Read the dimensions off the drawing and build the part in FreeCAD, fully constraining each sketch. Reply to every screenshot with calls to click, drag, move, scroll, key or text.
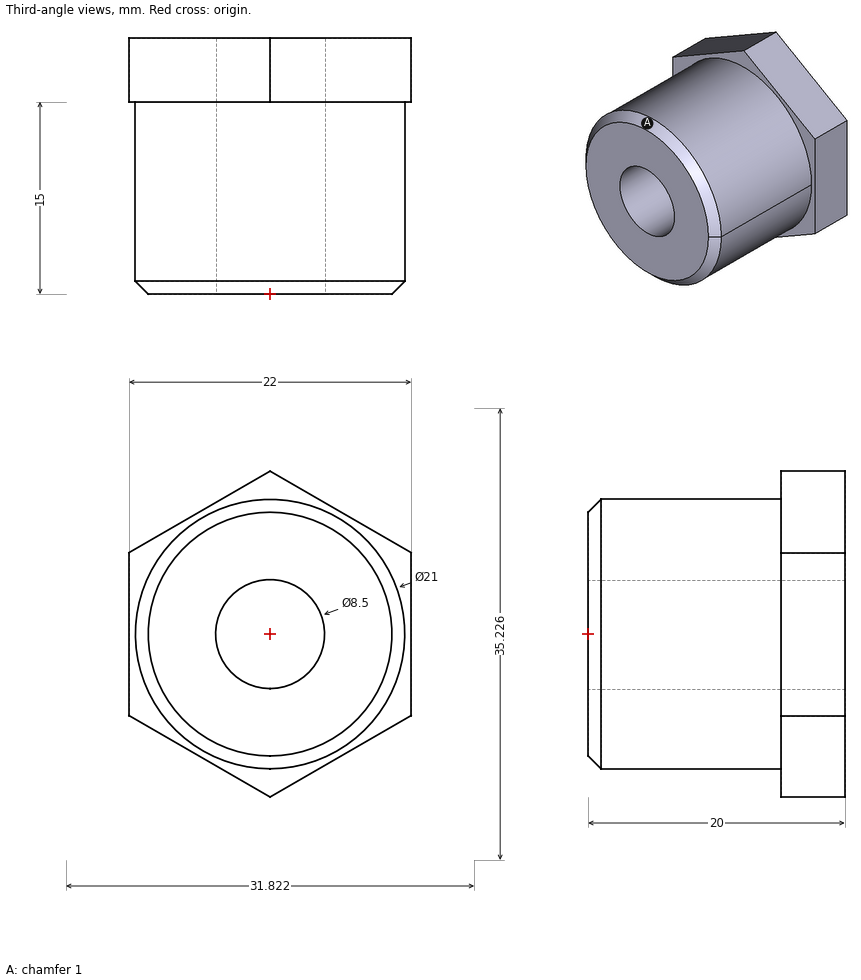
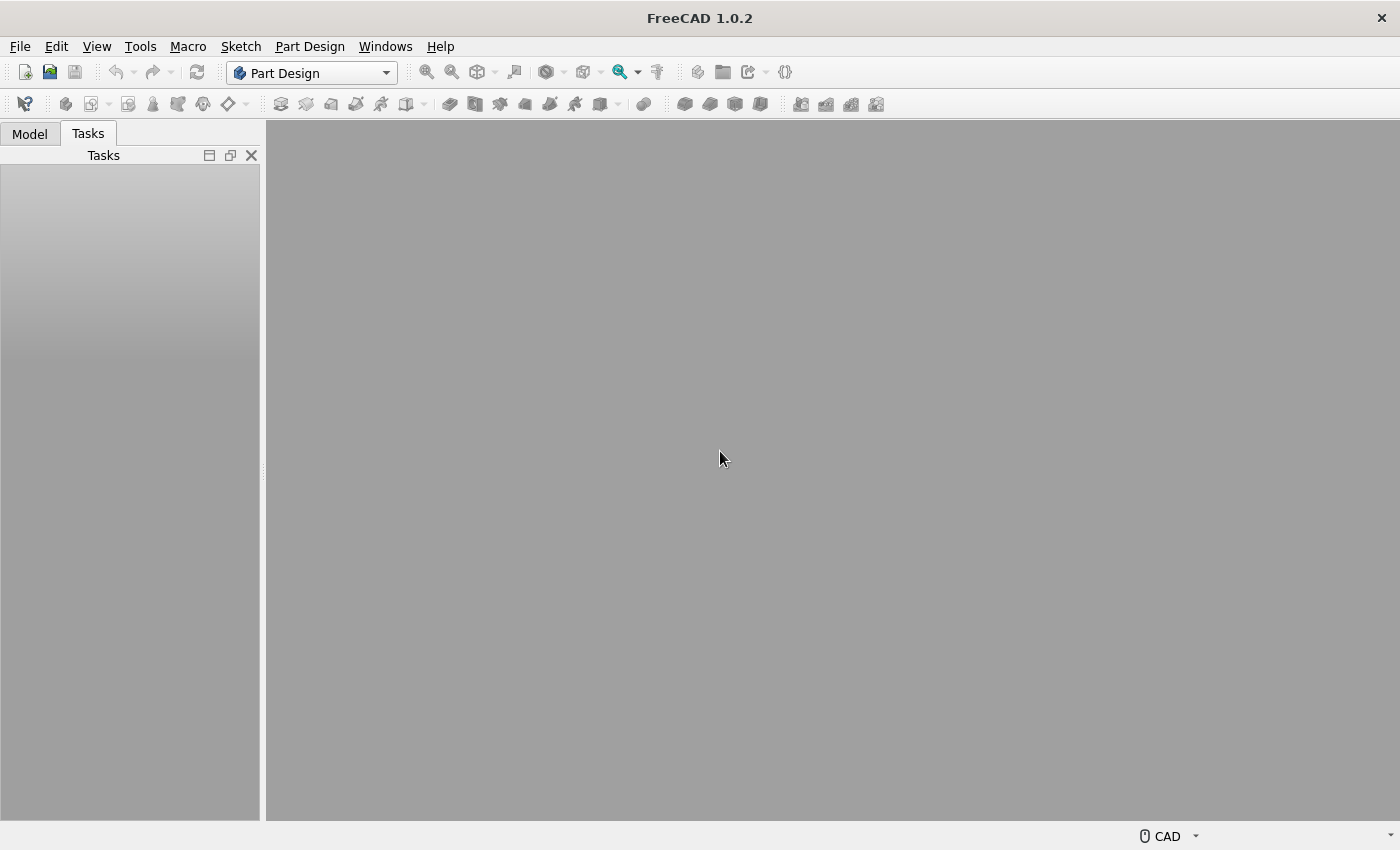
key(ctrl+n)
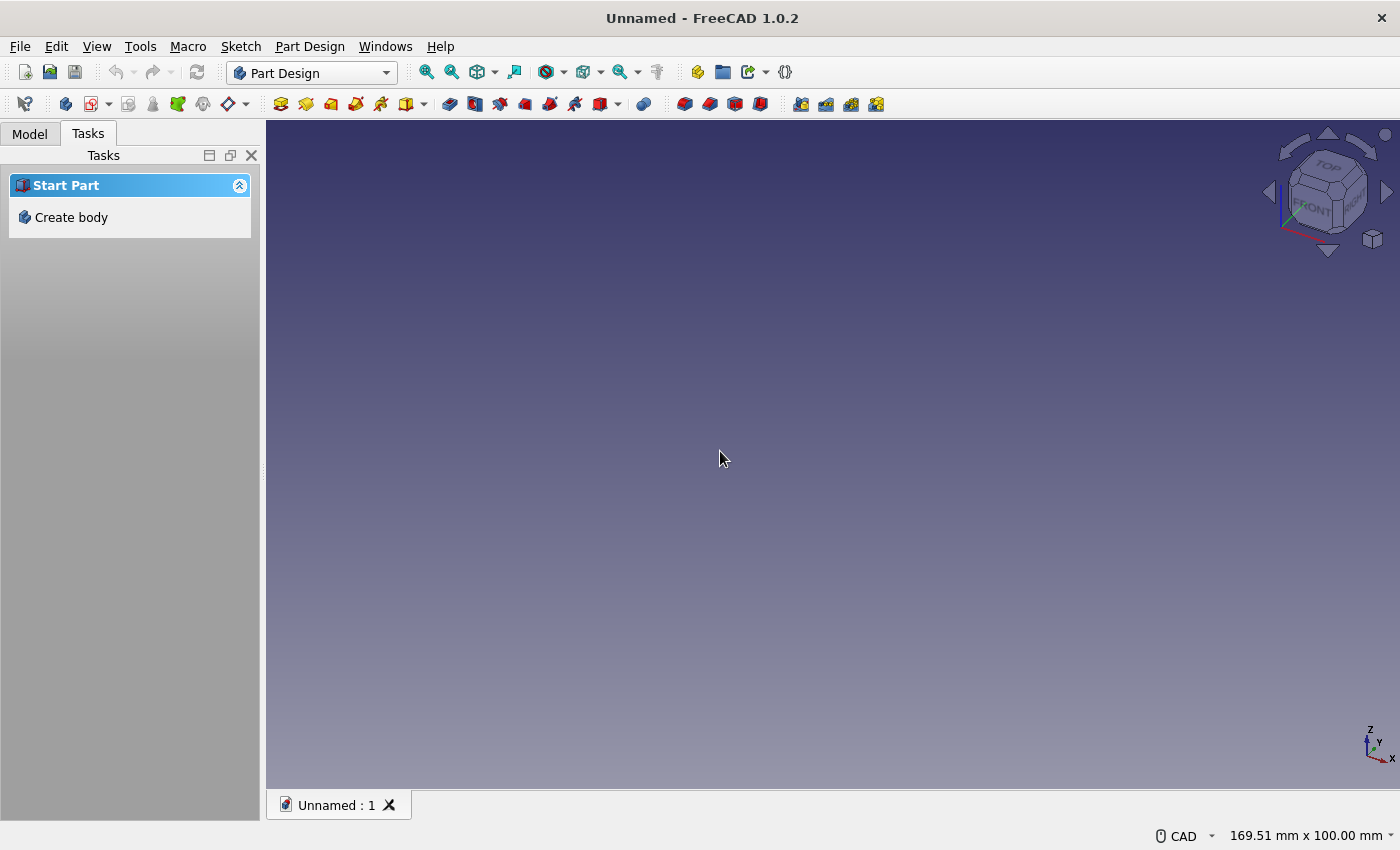
click(90, 104)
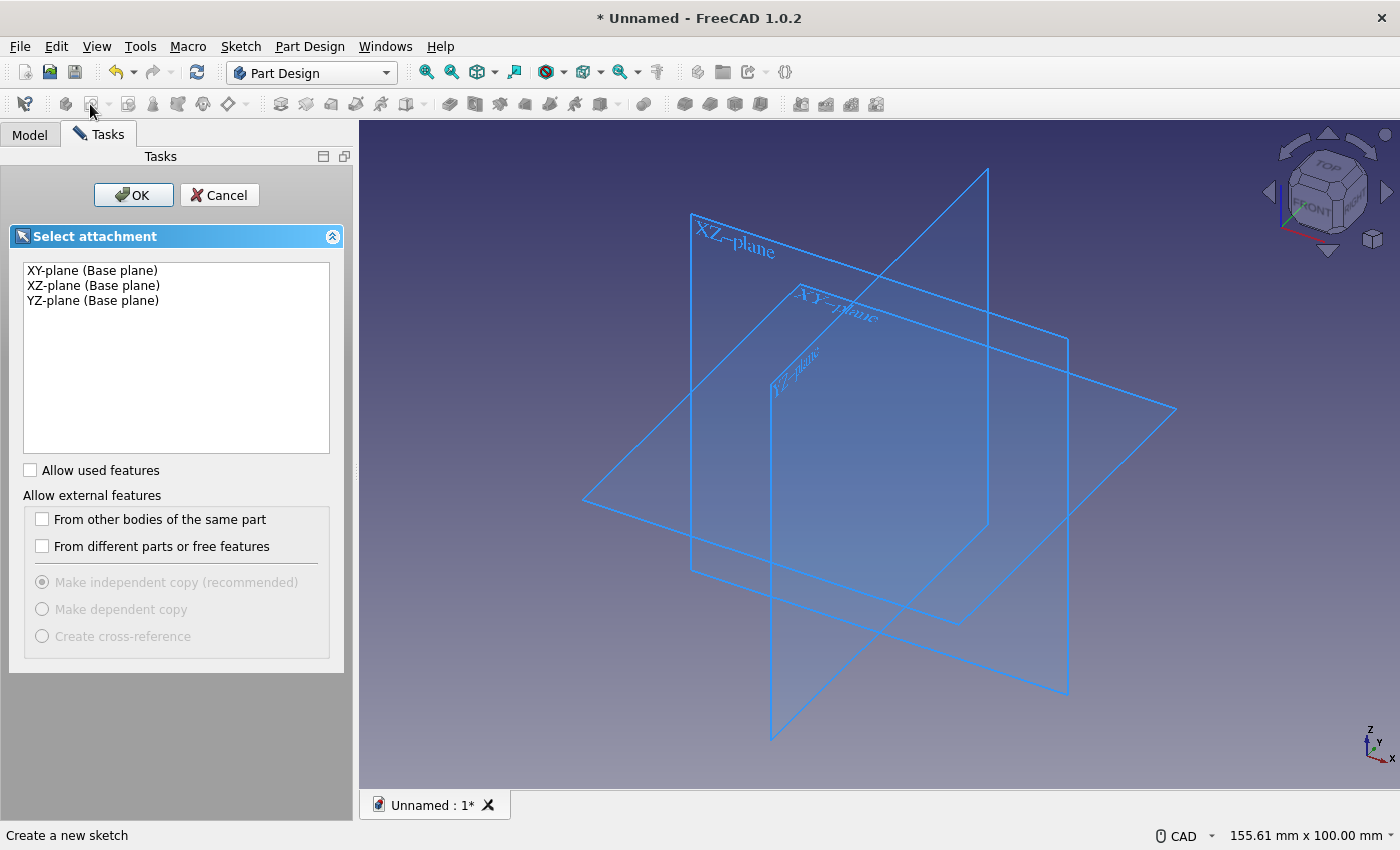
click(84, 286)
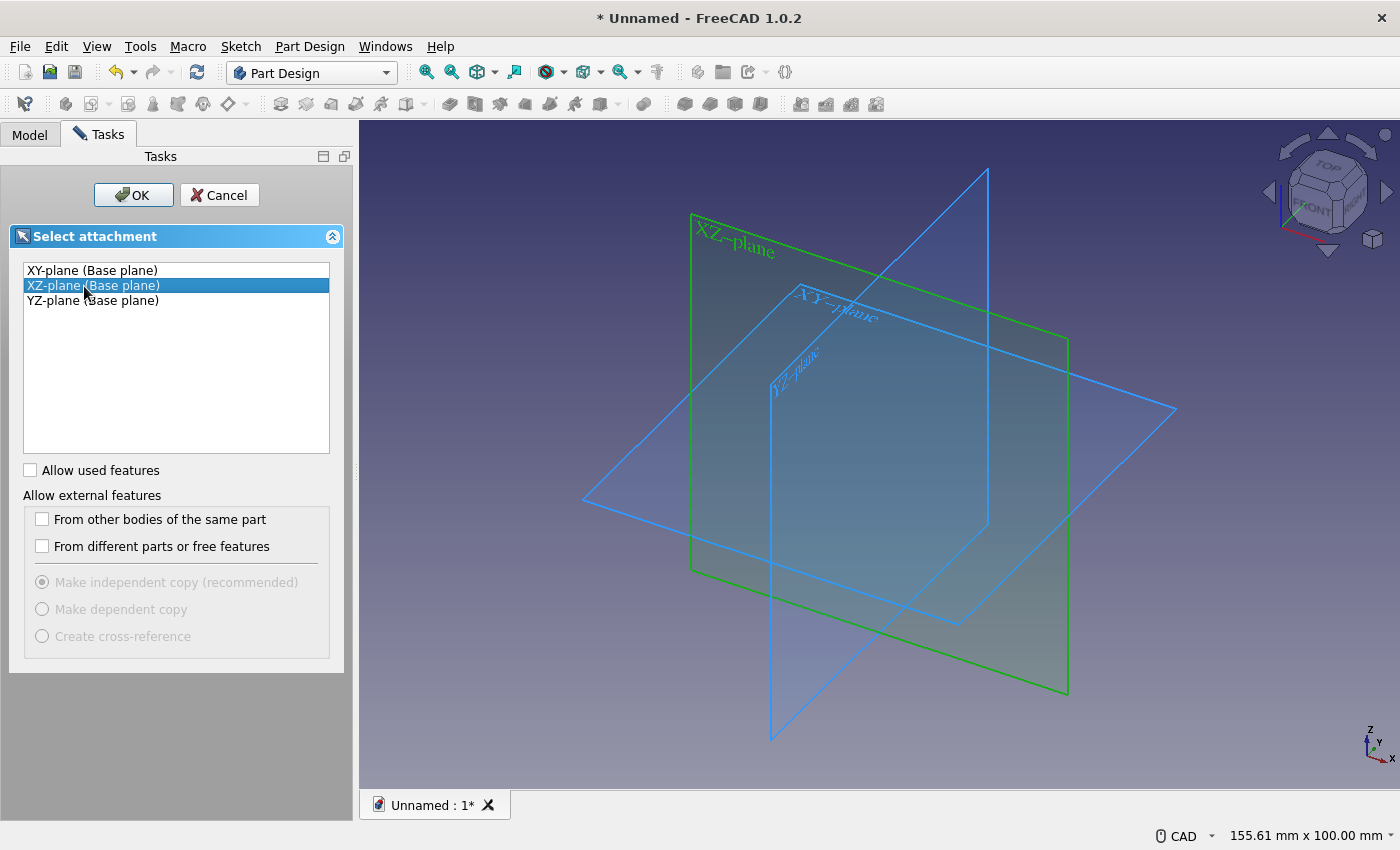
click(134, 195)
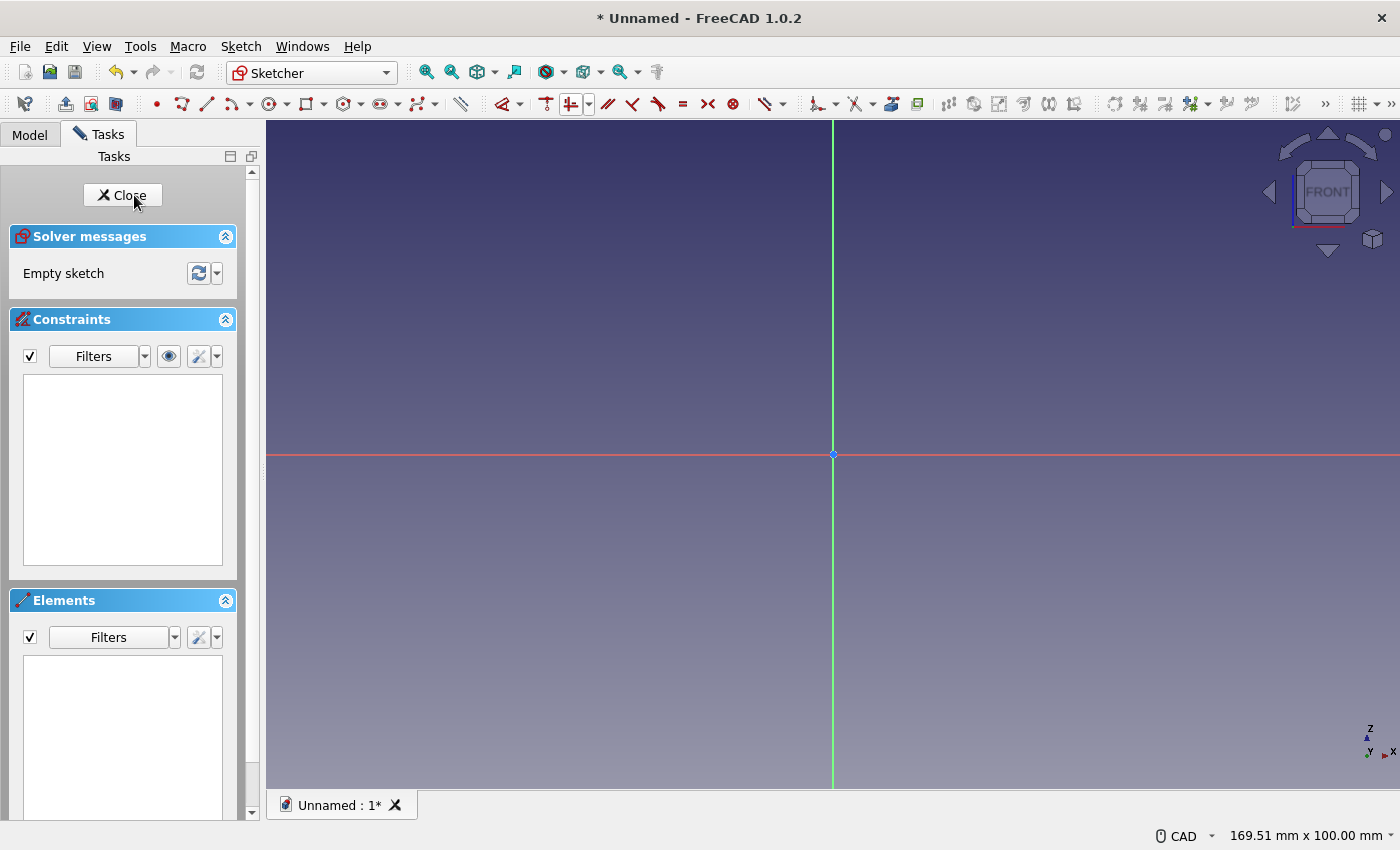
scroll(873, 454, up, 5)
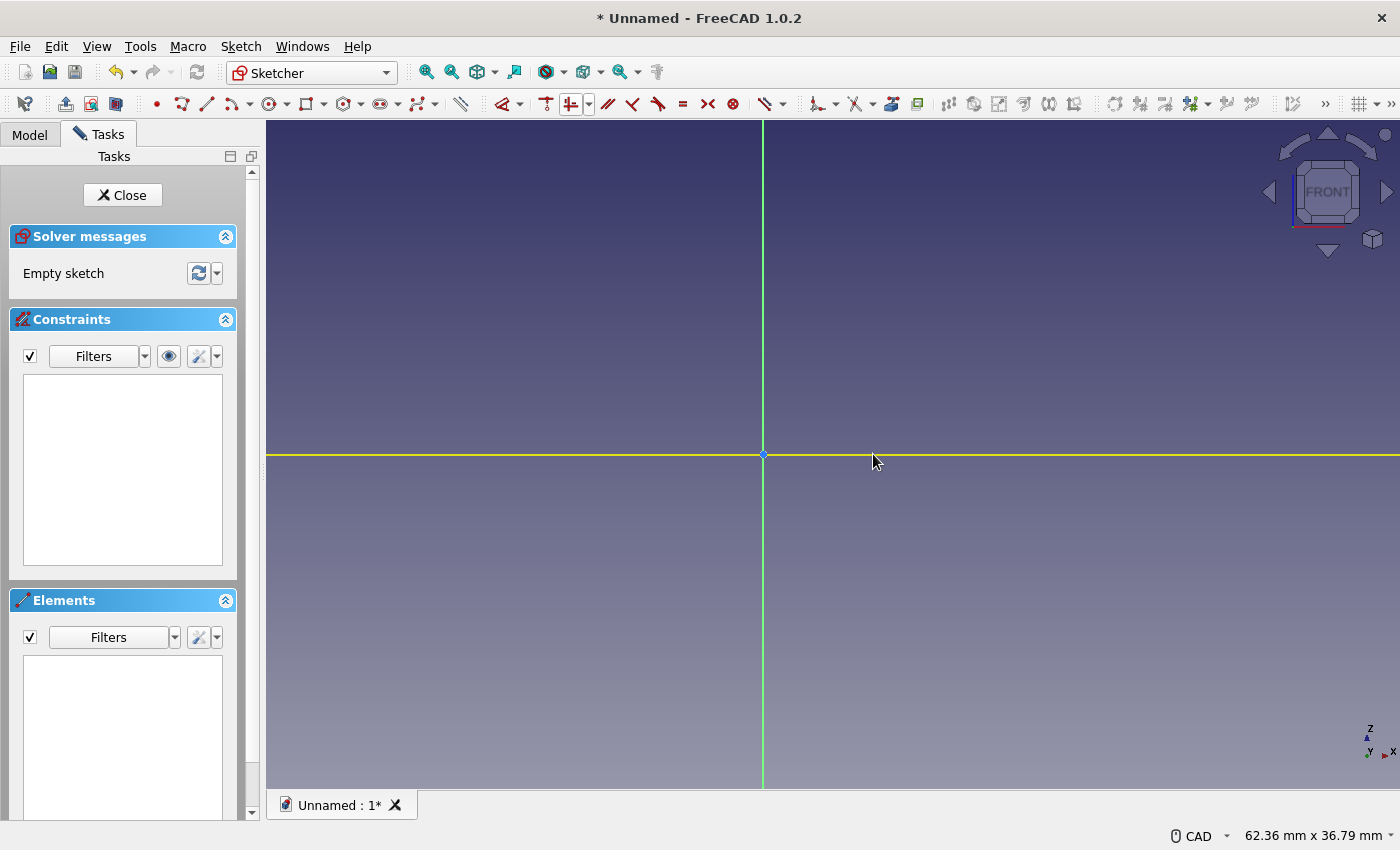
click(342, 104)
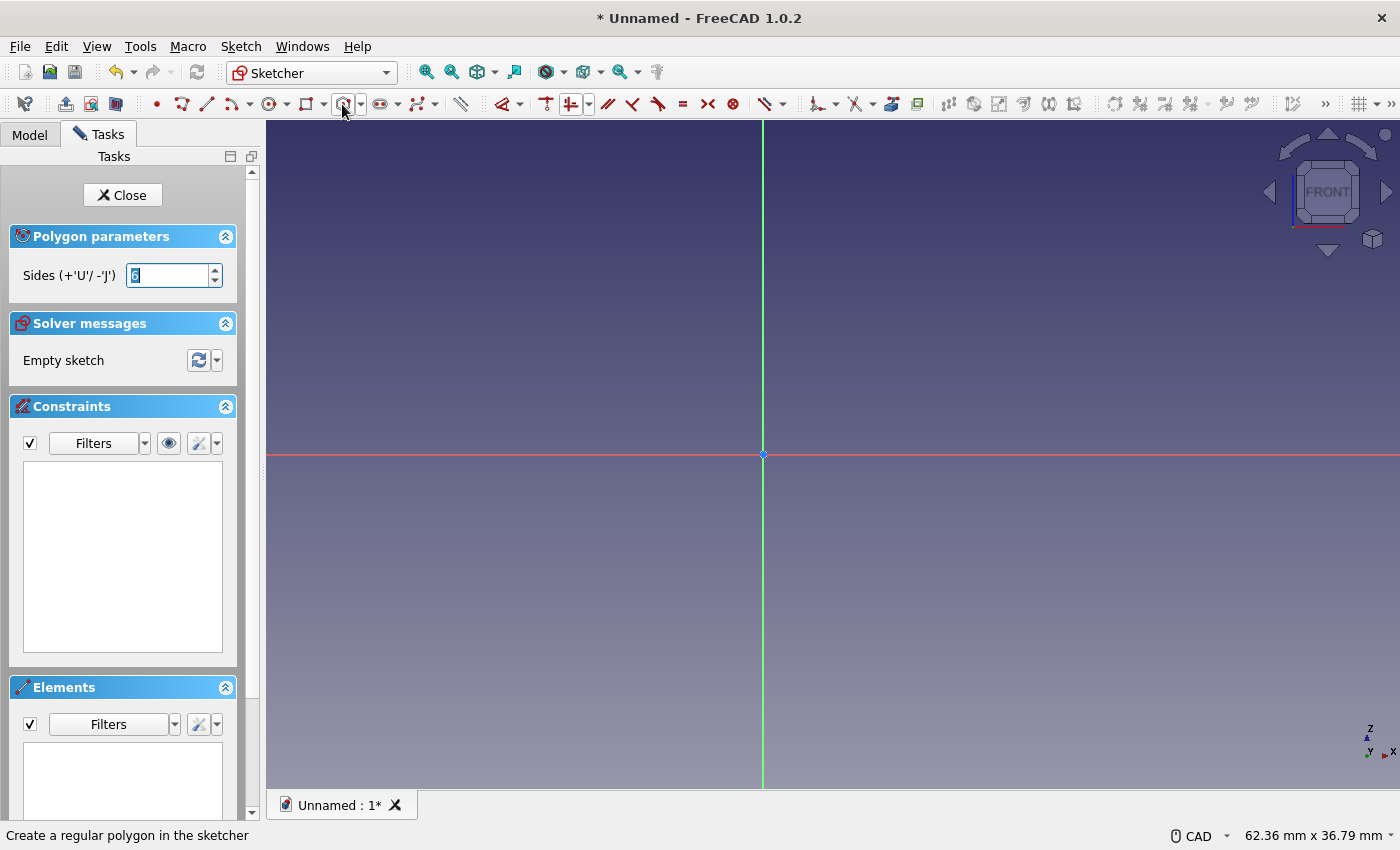
click(763, 454)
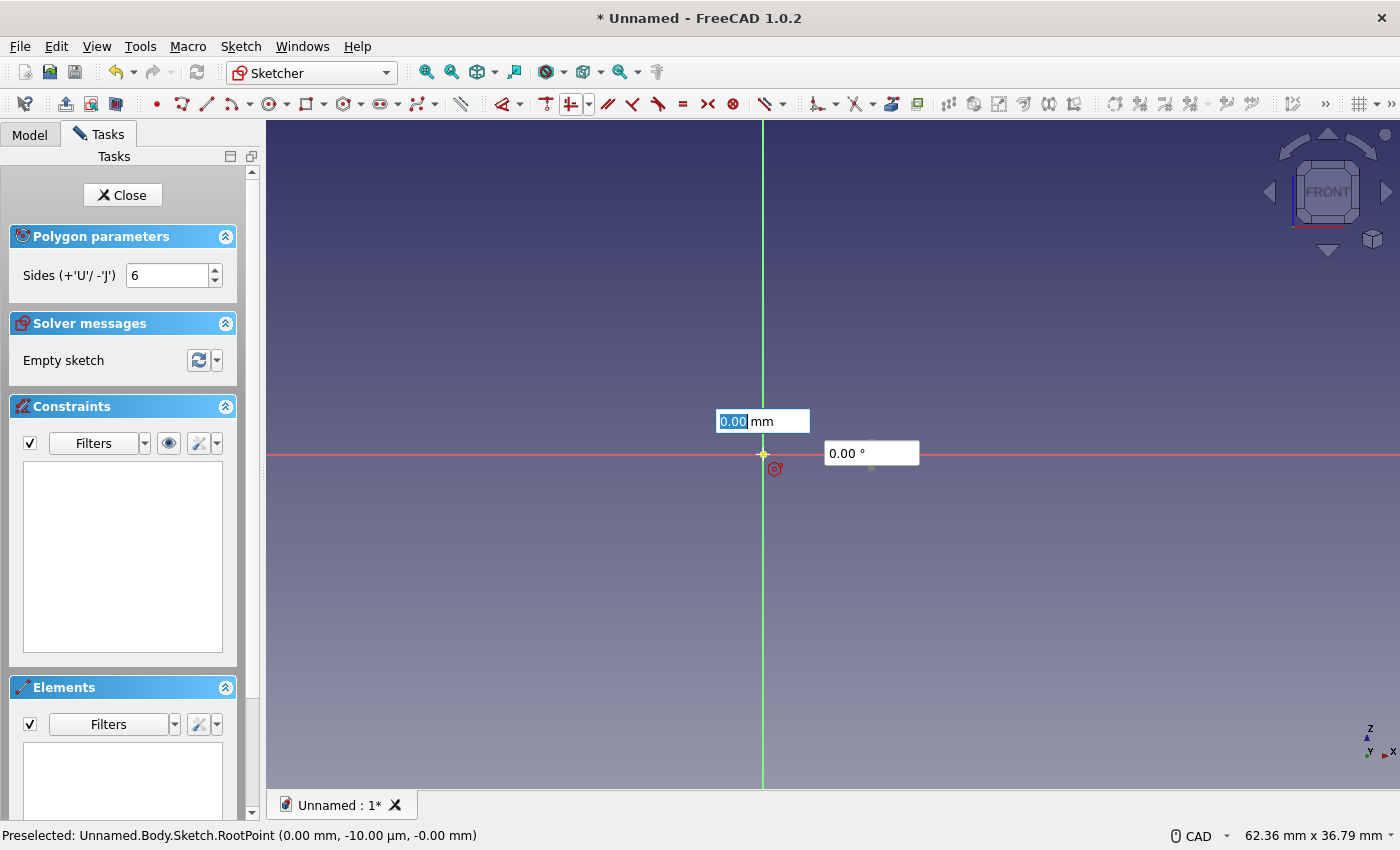
click(763, 685)
right_click(763, 685)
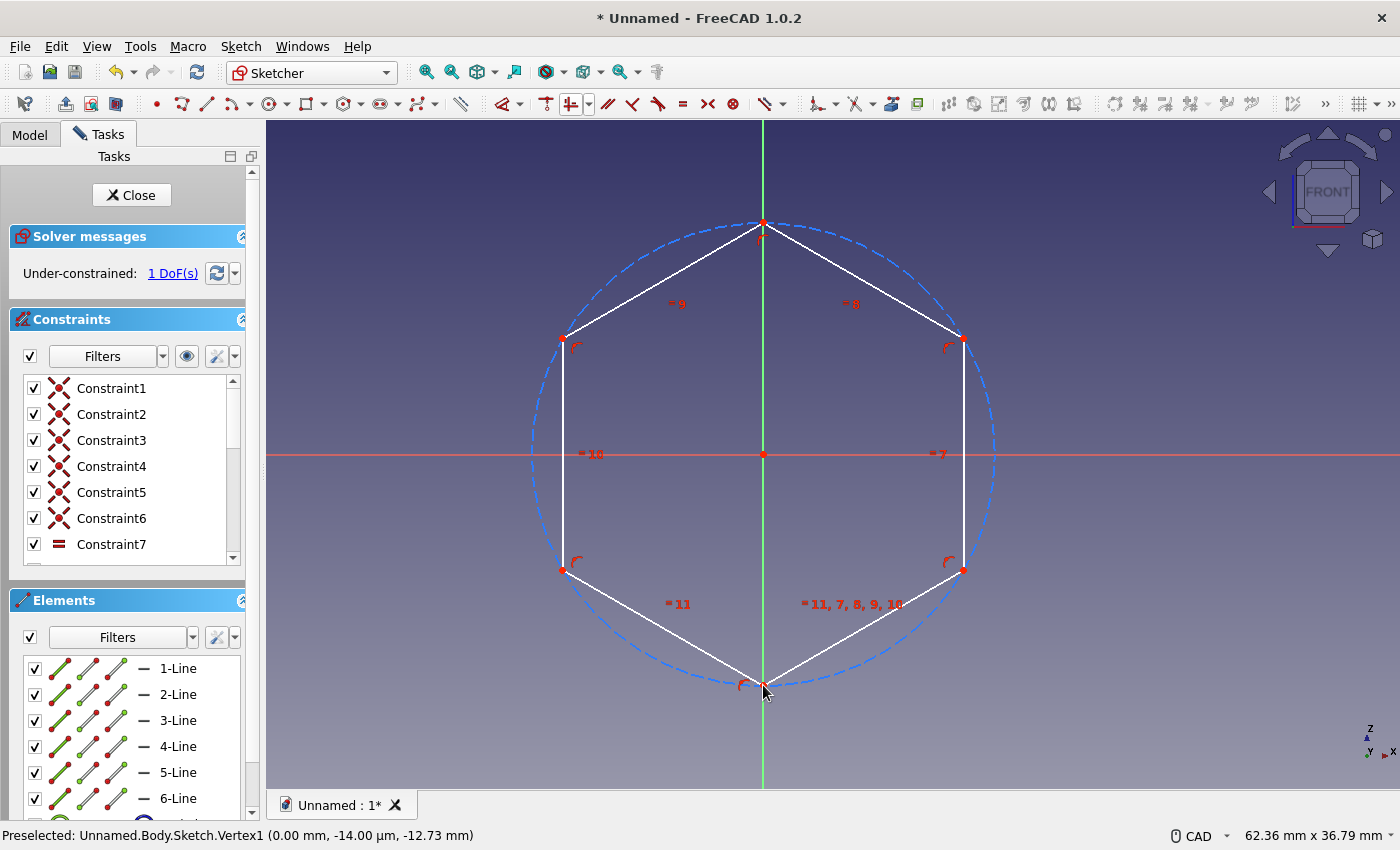
click(563, 339)